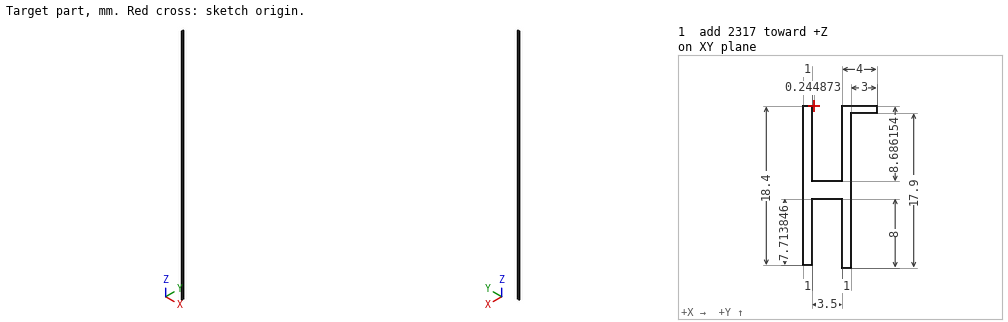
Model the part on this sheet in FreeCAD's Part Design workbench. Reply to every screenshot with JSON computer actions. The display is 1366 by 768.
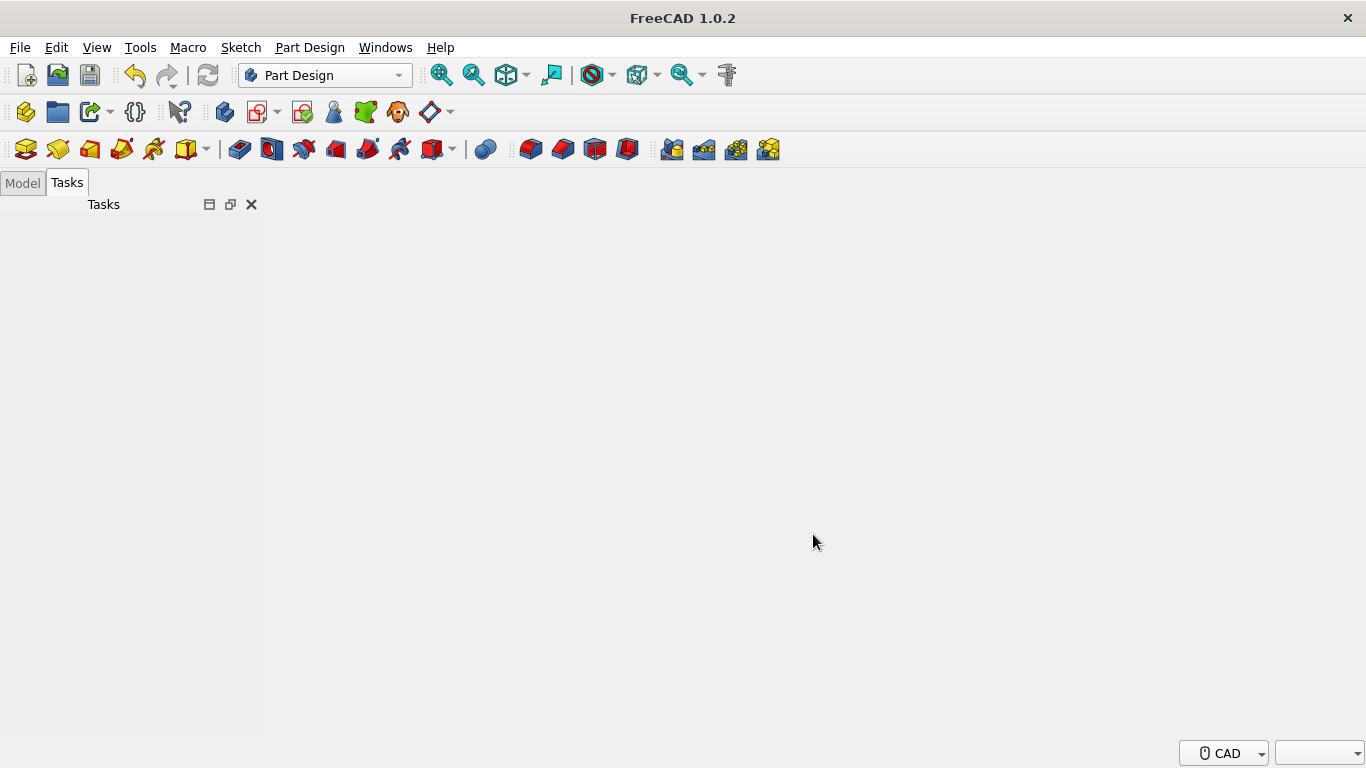
{"action": "key", "text": "ctrl+n"}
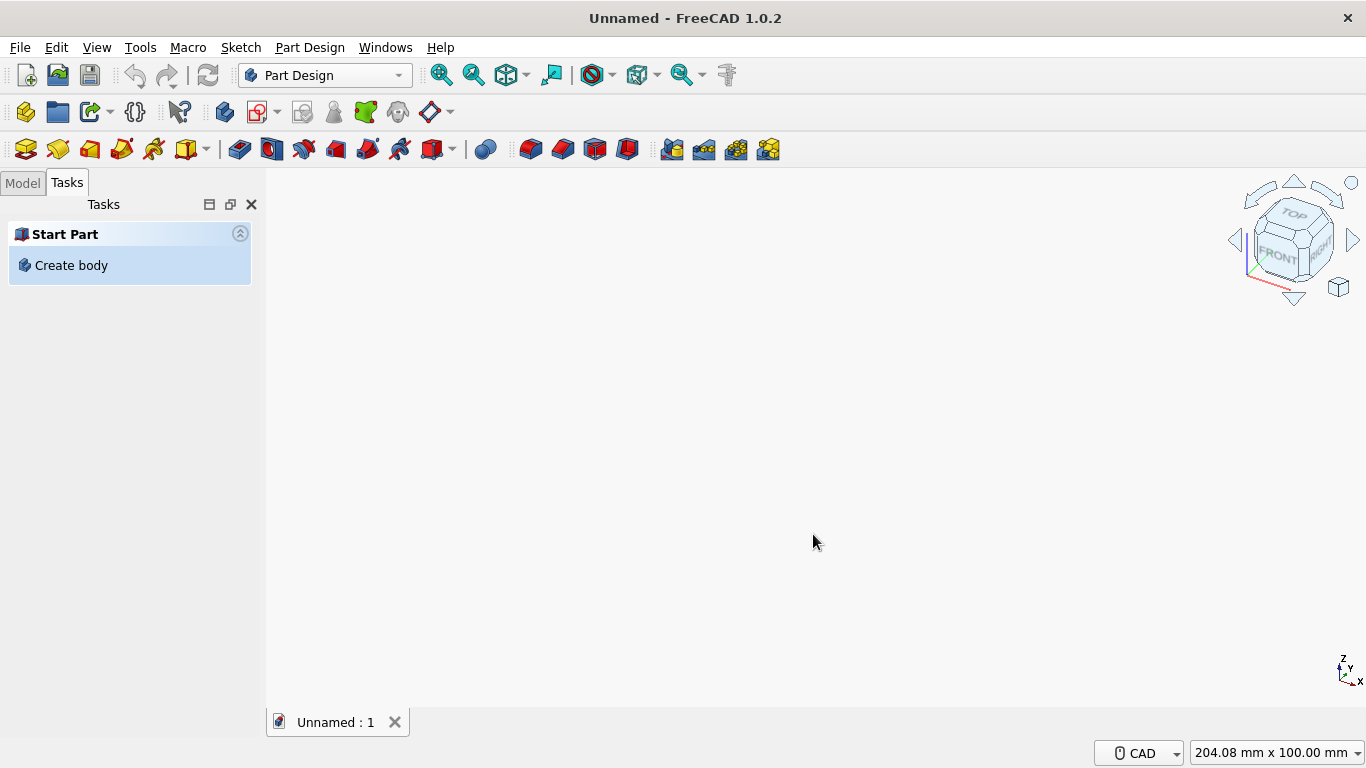
{"action": "left_click", "coordinate": [258, 112]}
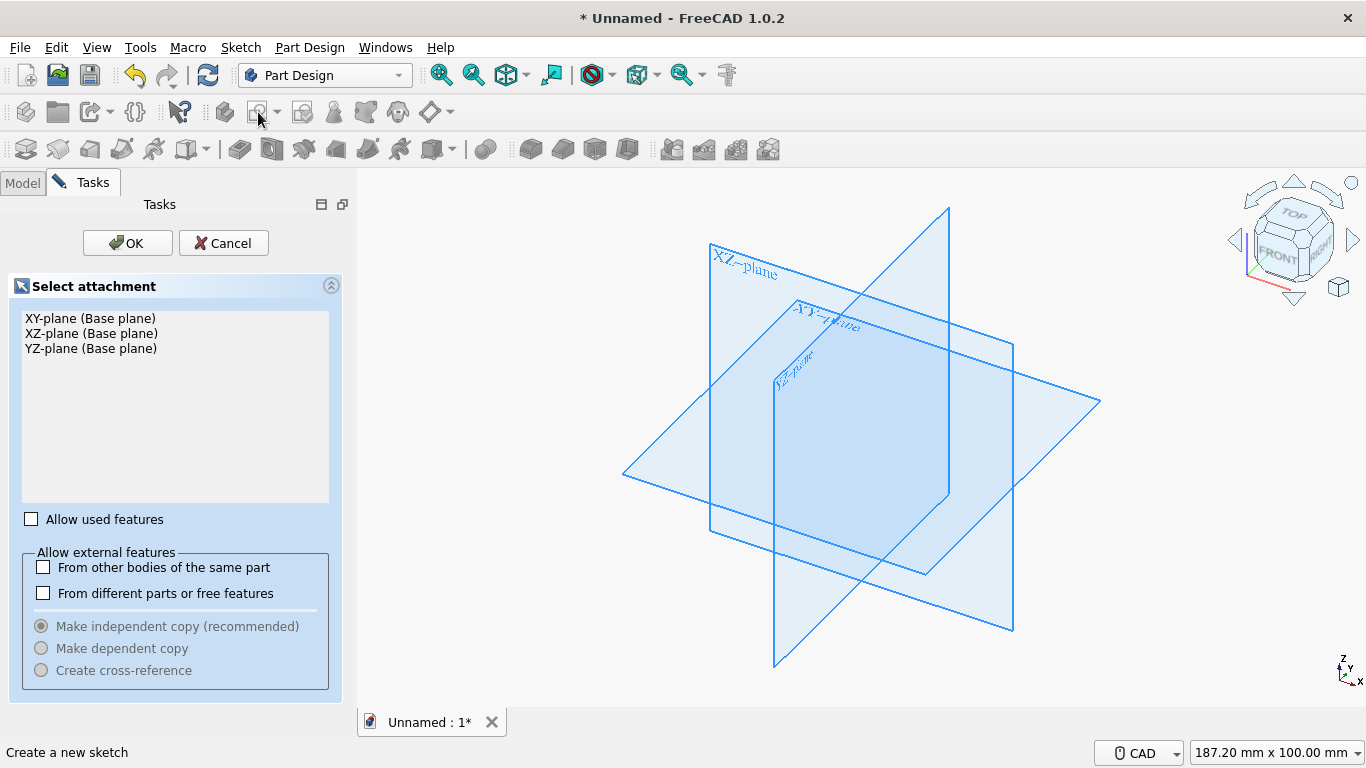
{"action": "left_click", "coordinate": [82, 318]}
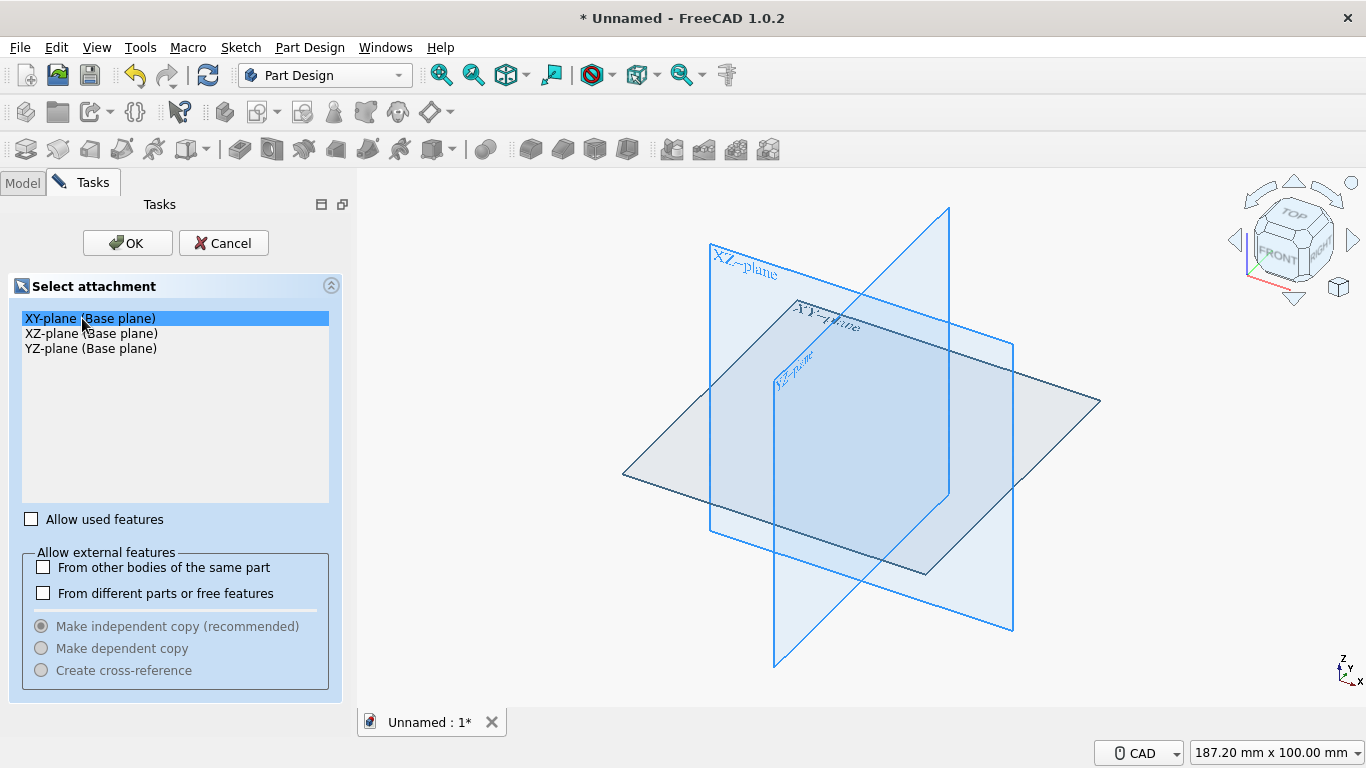
{"action": "left_click", "coordinate": [128, 243]}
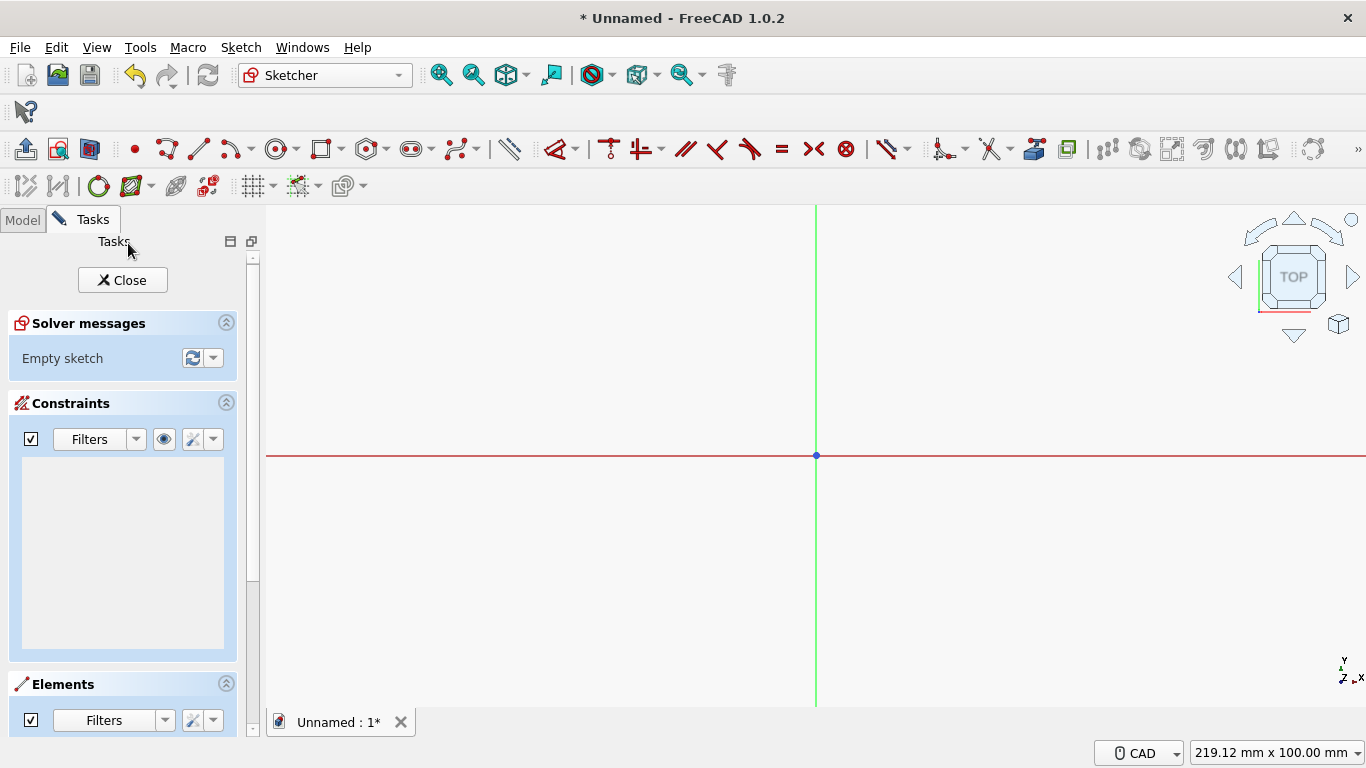
{"action": "scroll", "coordinate": [867, 523], "scroll_direction": "up", "scroll_amount": 6}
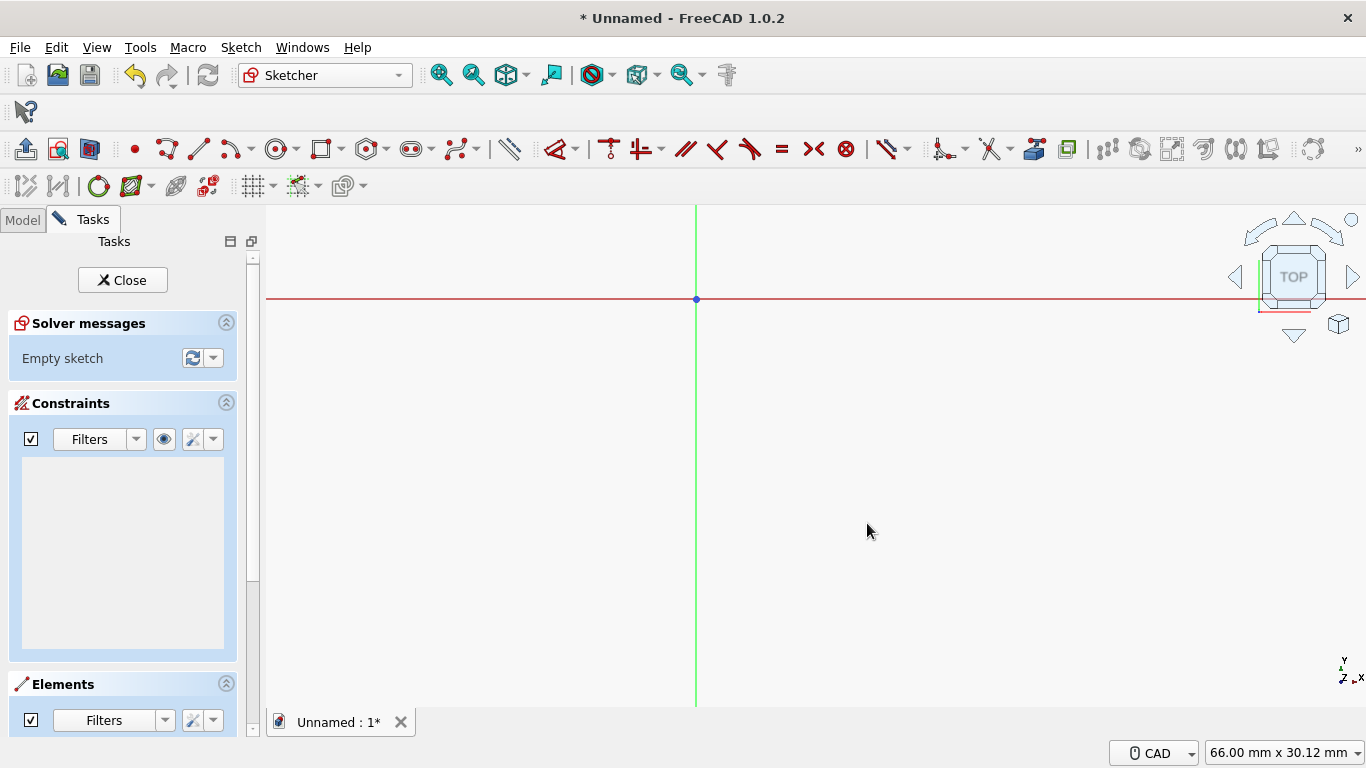
{"action": "left_click", "coordinate": [168, 150]}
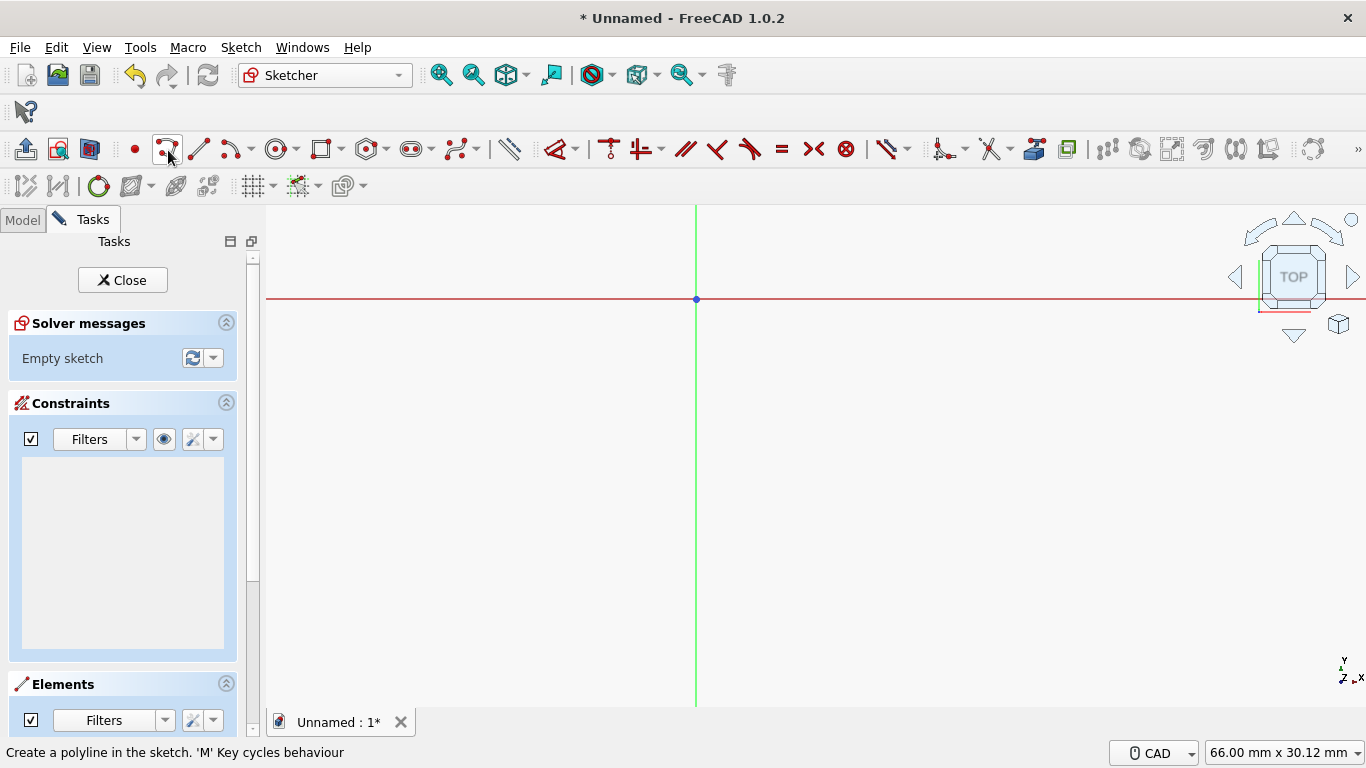
{"action": "scroll", "coordinate": [692, 299], "scroll_direction": "up", "scroll_amount": 7}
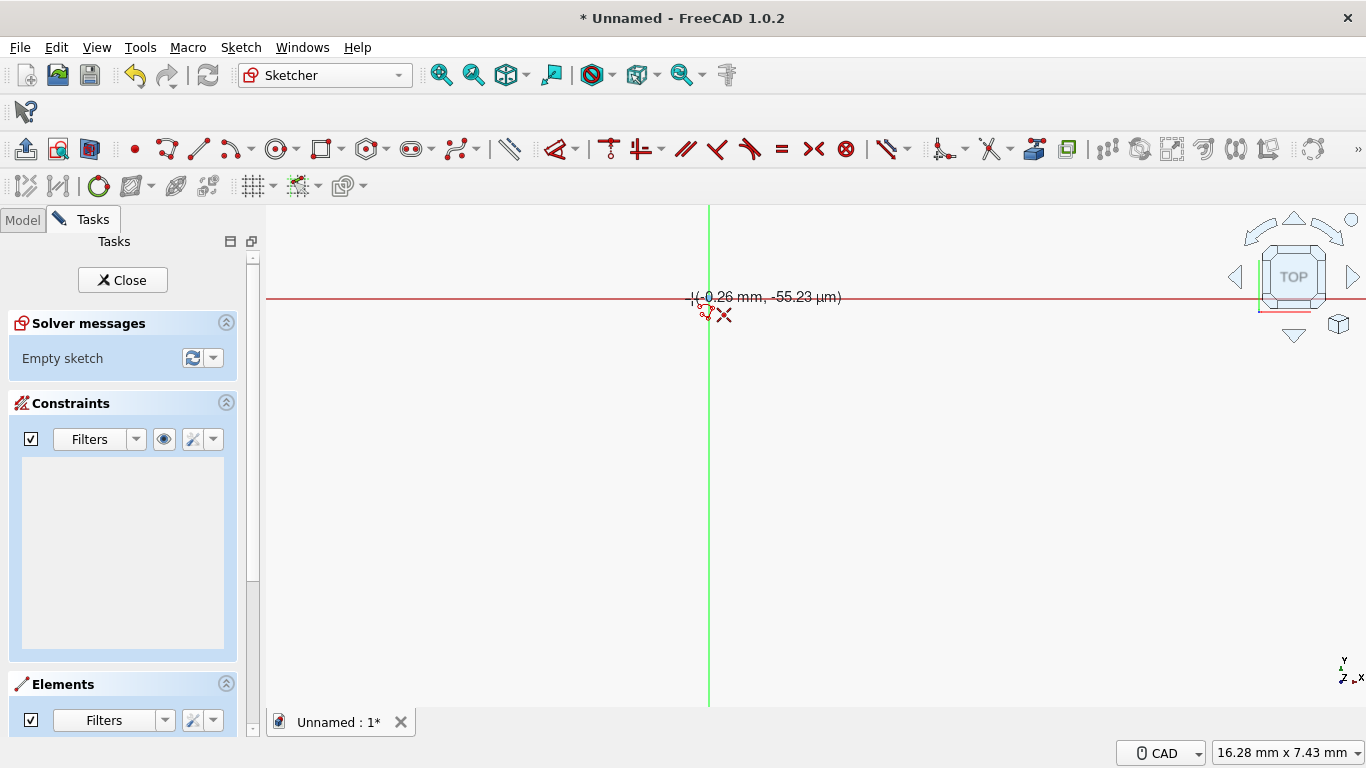
{"action": "left_click", "coordinate": [692, 299]}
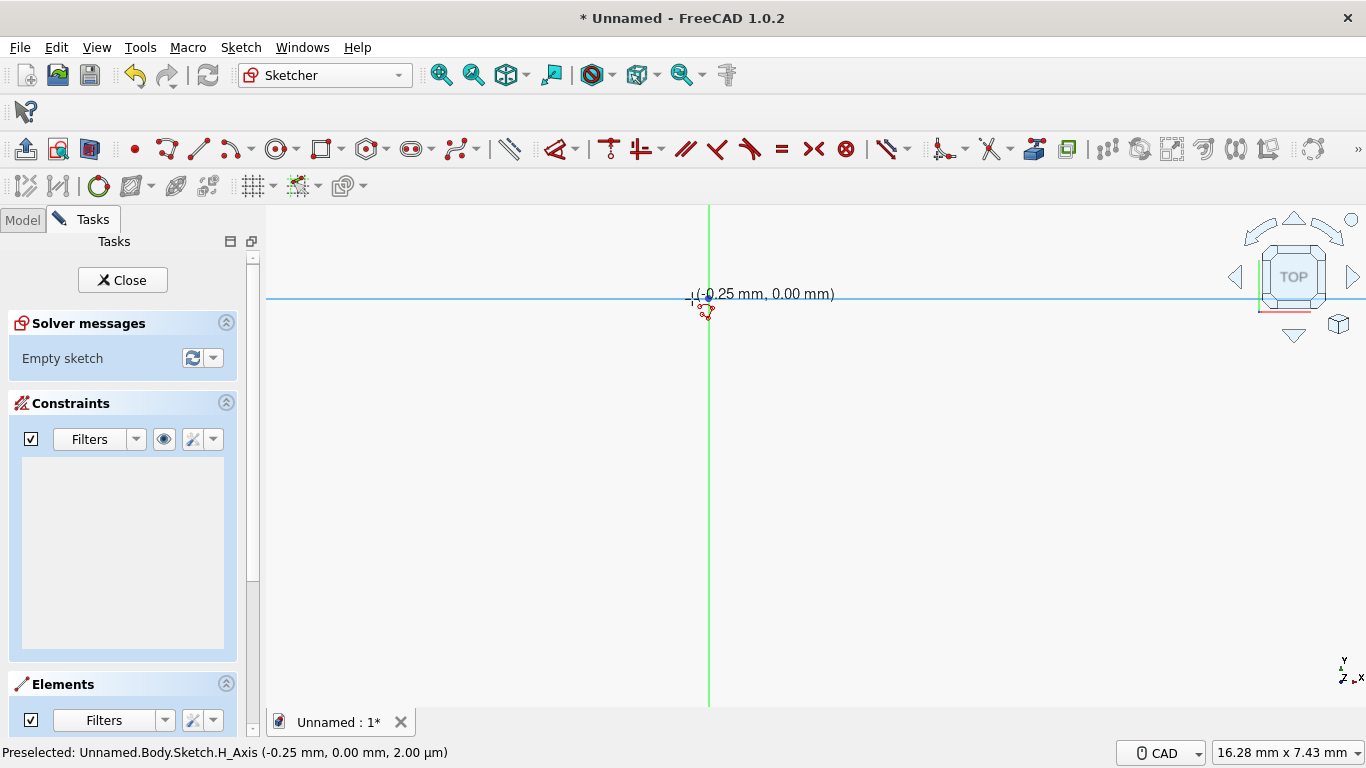
{"action": "scroll", "coordinate": [694, 301], "scroll_direction": "down", "scroll_amount": 7}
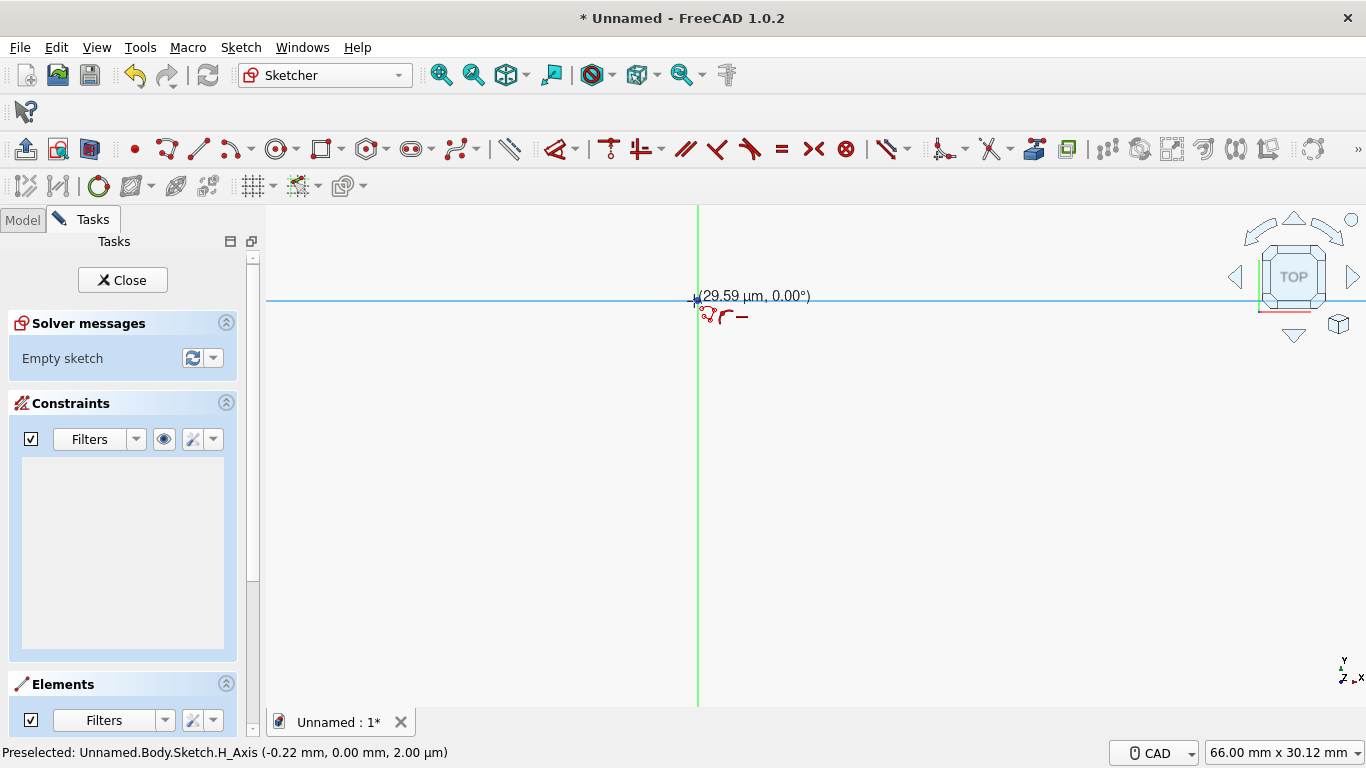
{"action": "left_click", "coordinate": [677, 310]}
{"action": "left_click", "coordinate": [677, 607]}